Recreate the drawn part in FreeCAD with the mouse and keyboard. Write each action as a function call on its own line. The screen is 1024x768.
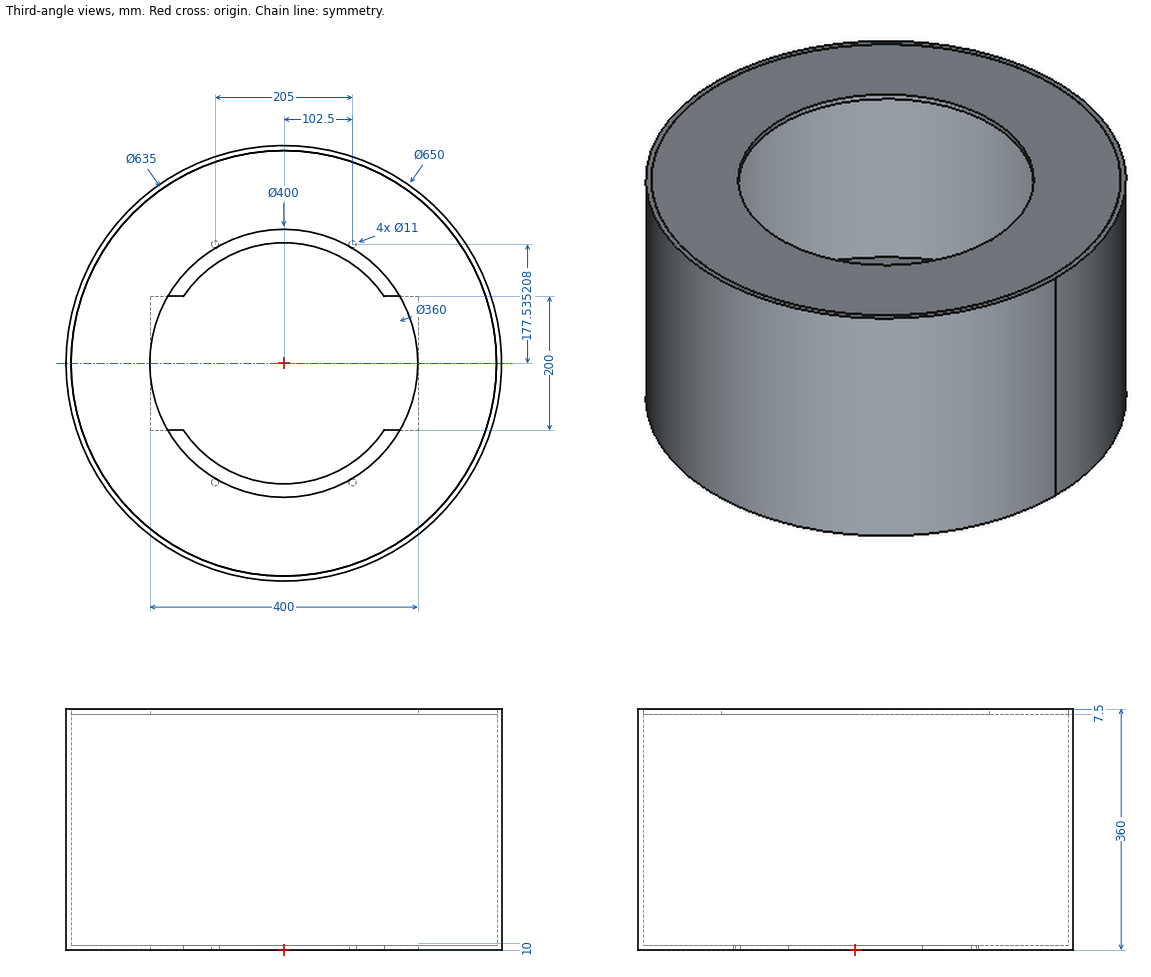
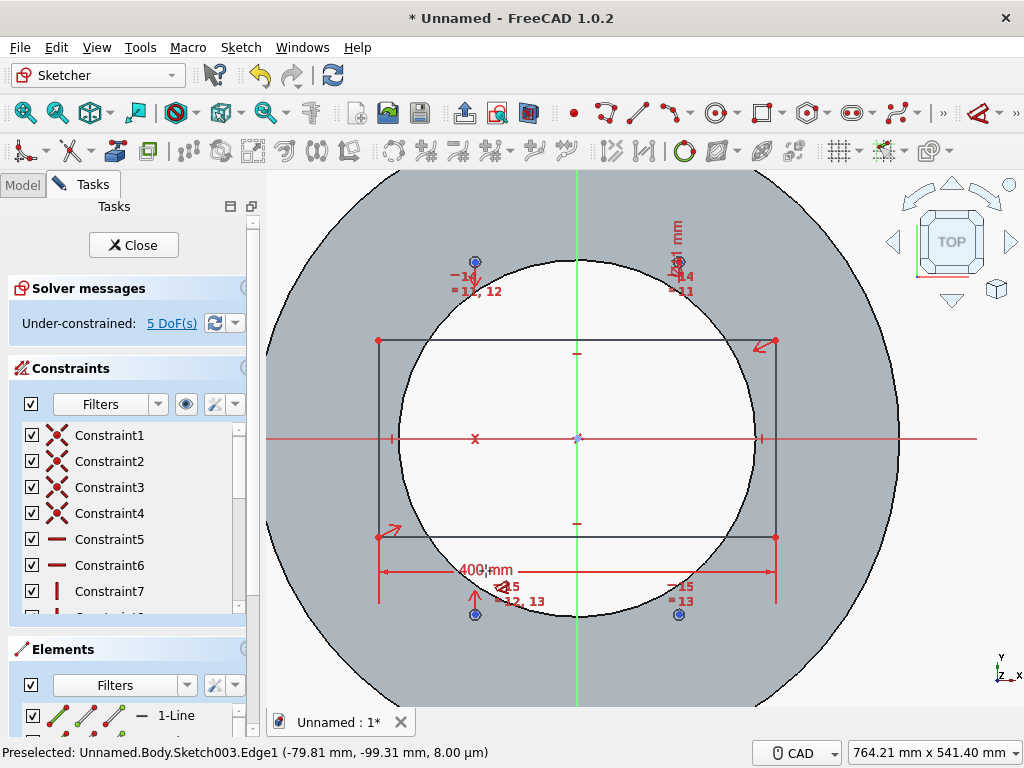
click(776, 478)
click(810, 393)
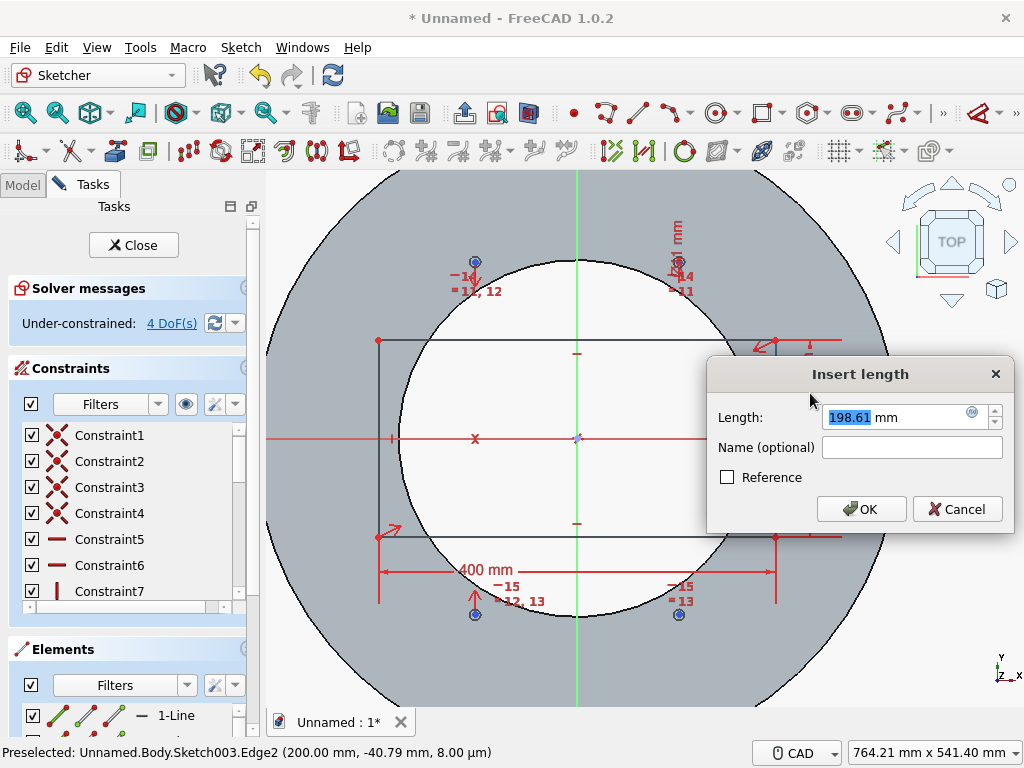
text(200)
key(Return)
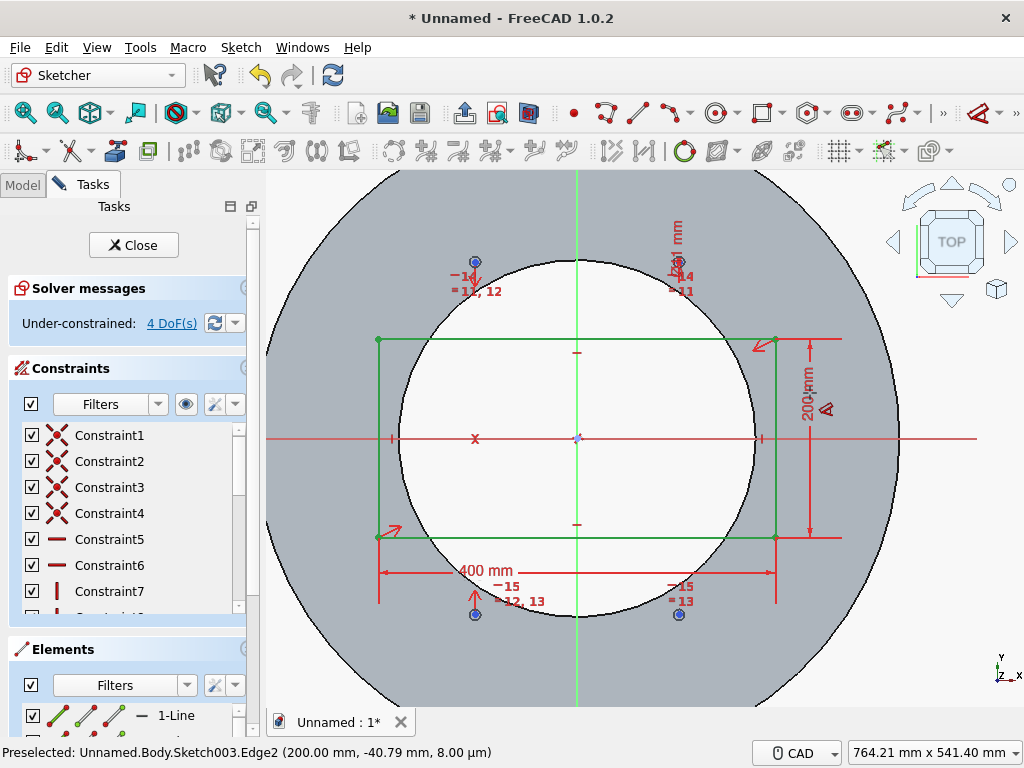
click(679, 262)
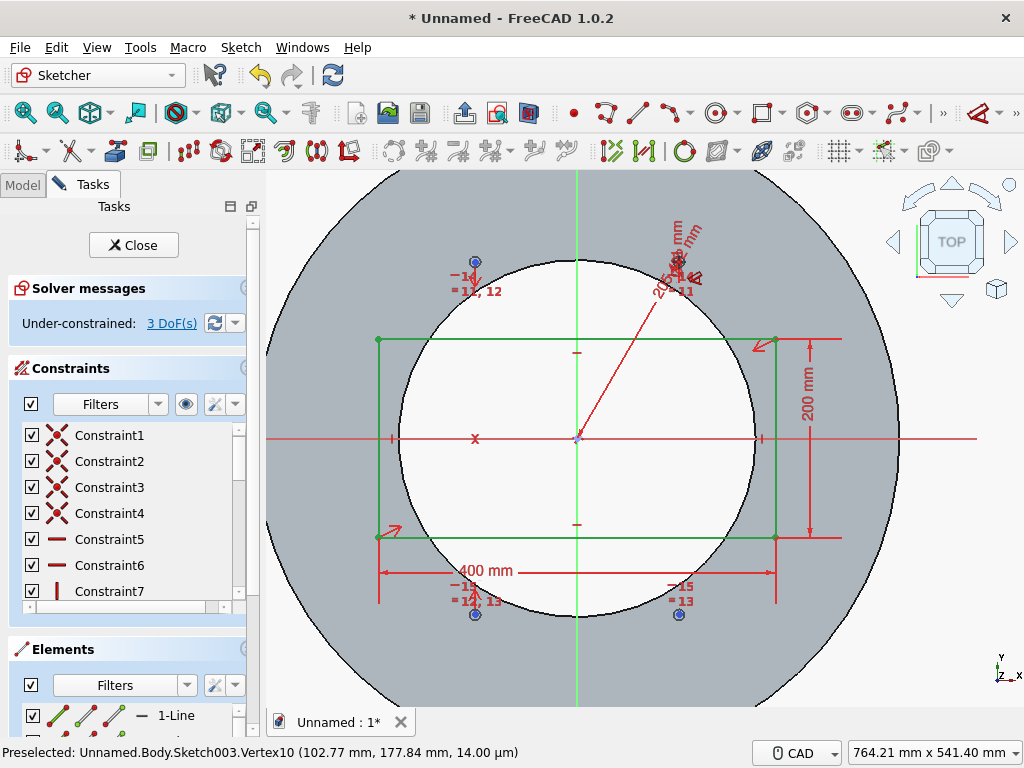
click(475, 262)
click(530, 228)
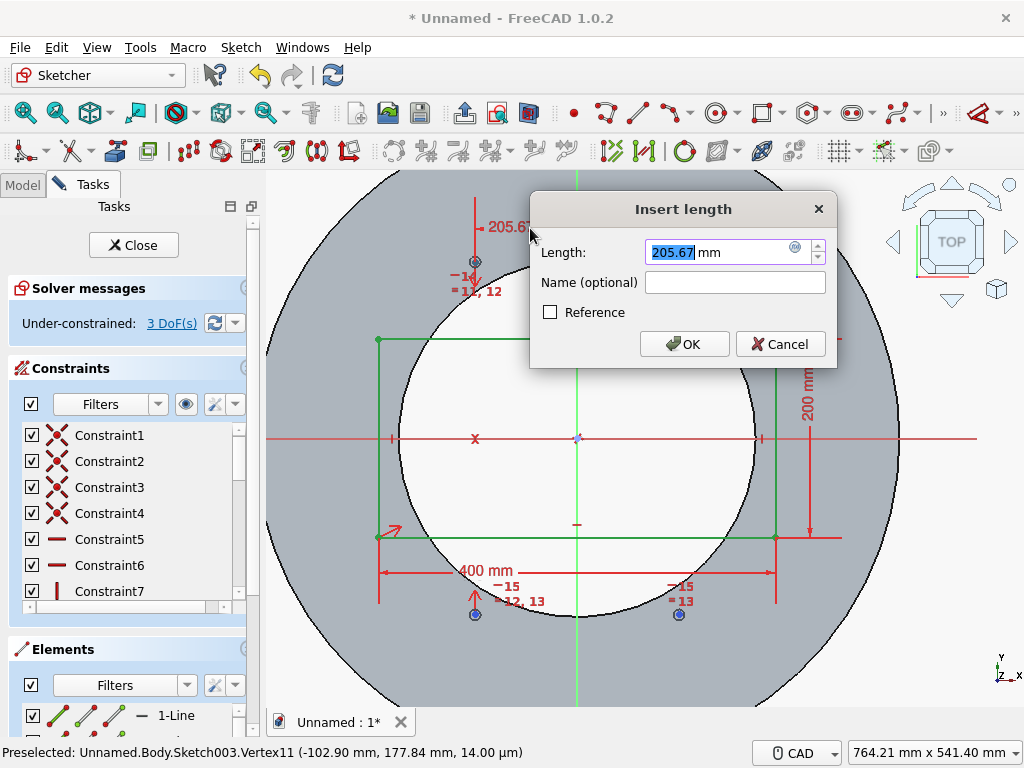
text(205)
key(Return)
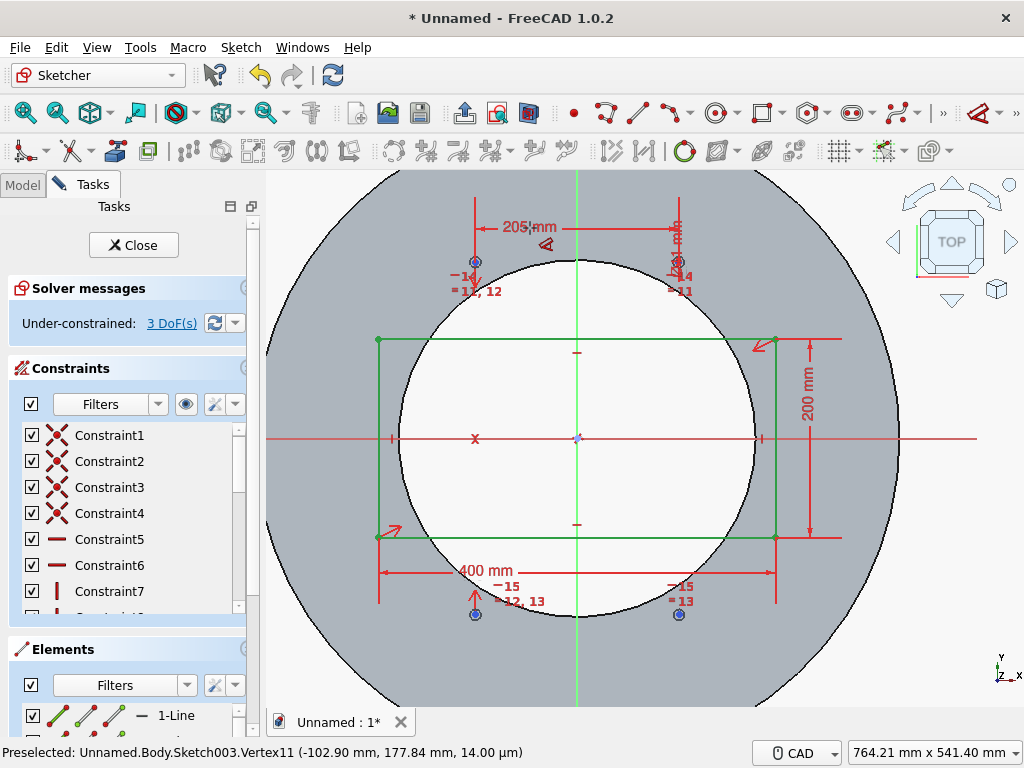
click(475, 615)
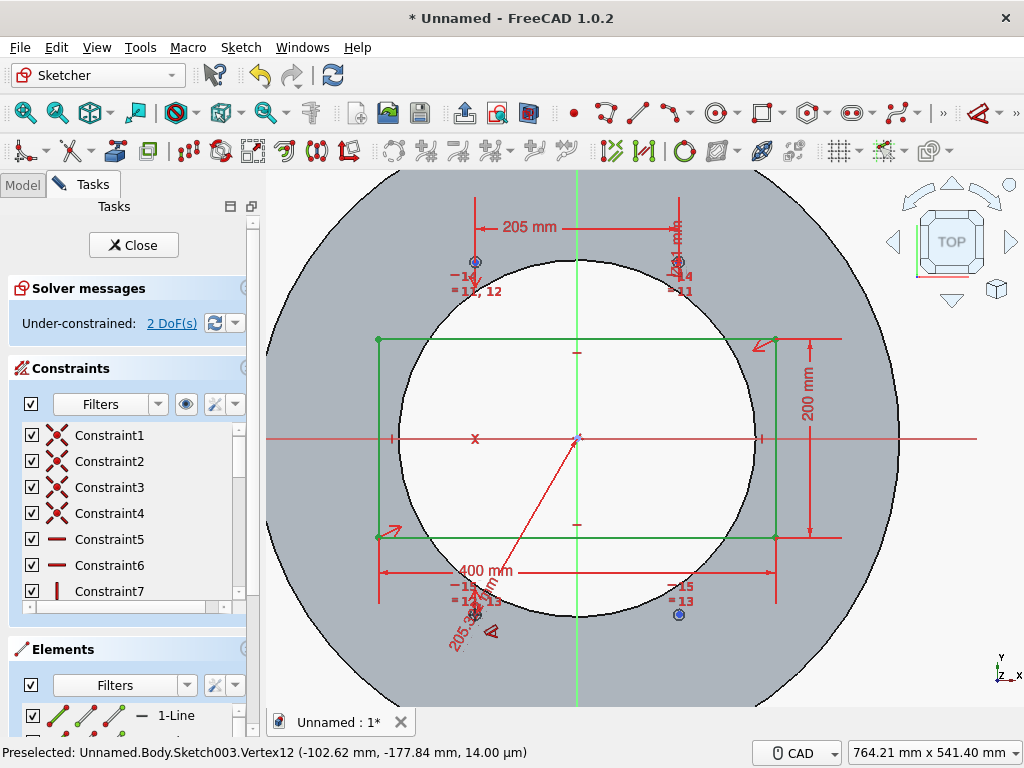
click(679, 615)
click(530, 649)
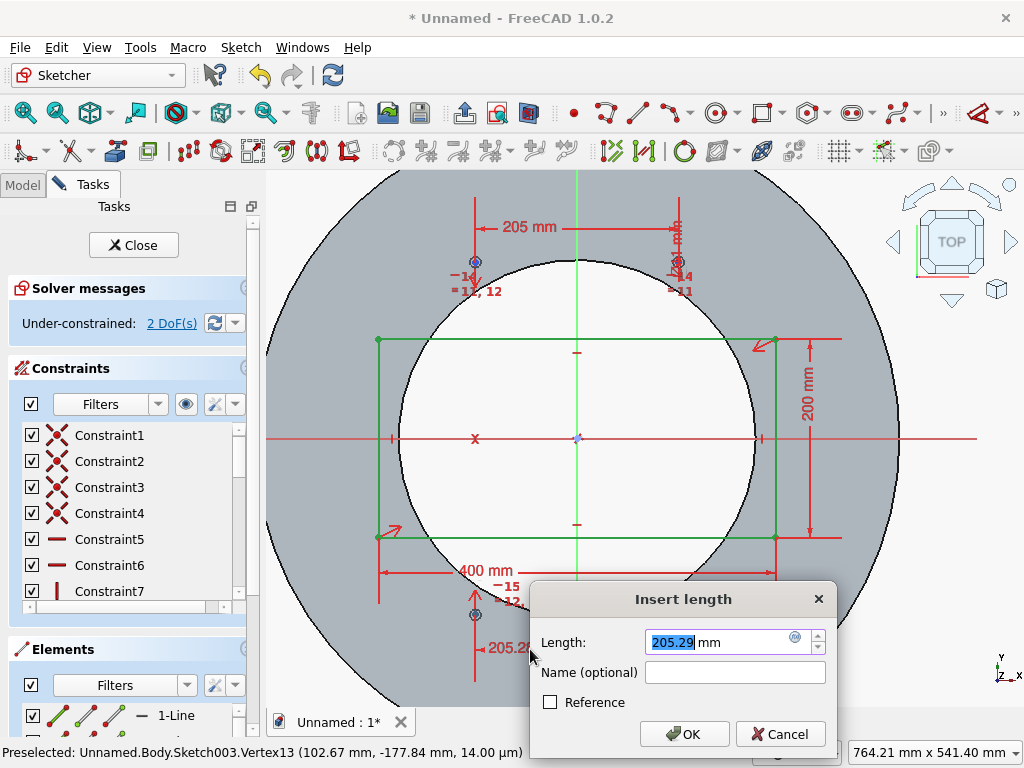
text(205)
key(Return)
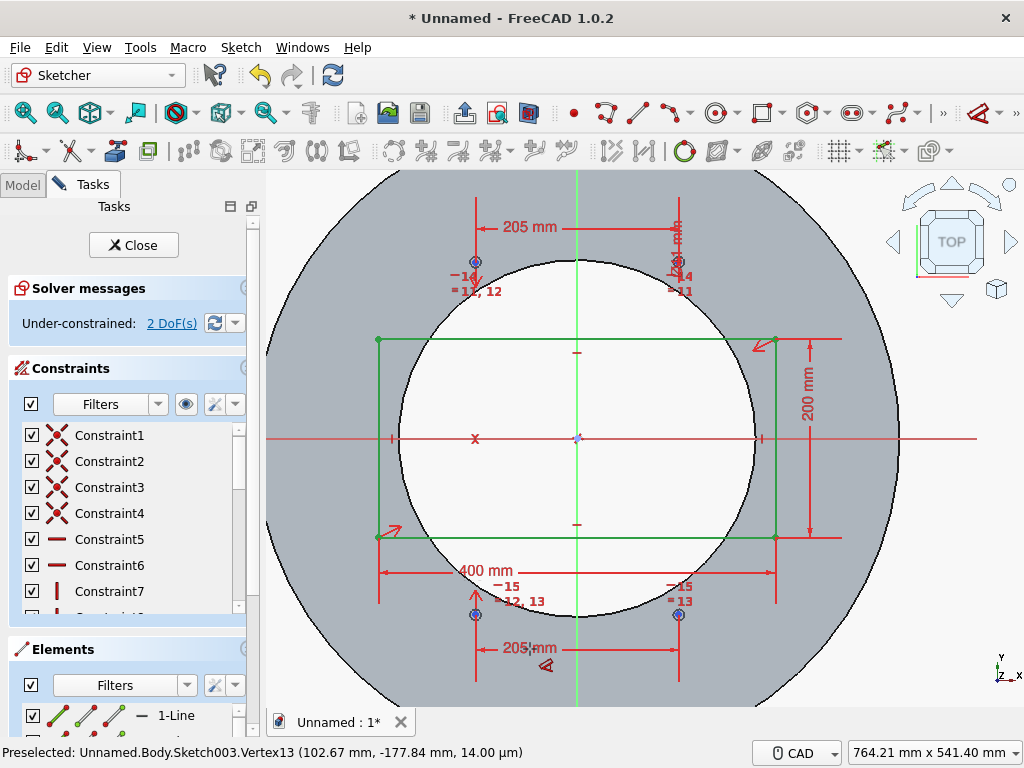
click(679, 262)
click(628, 228)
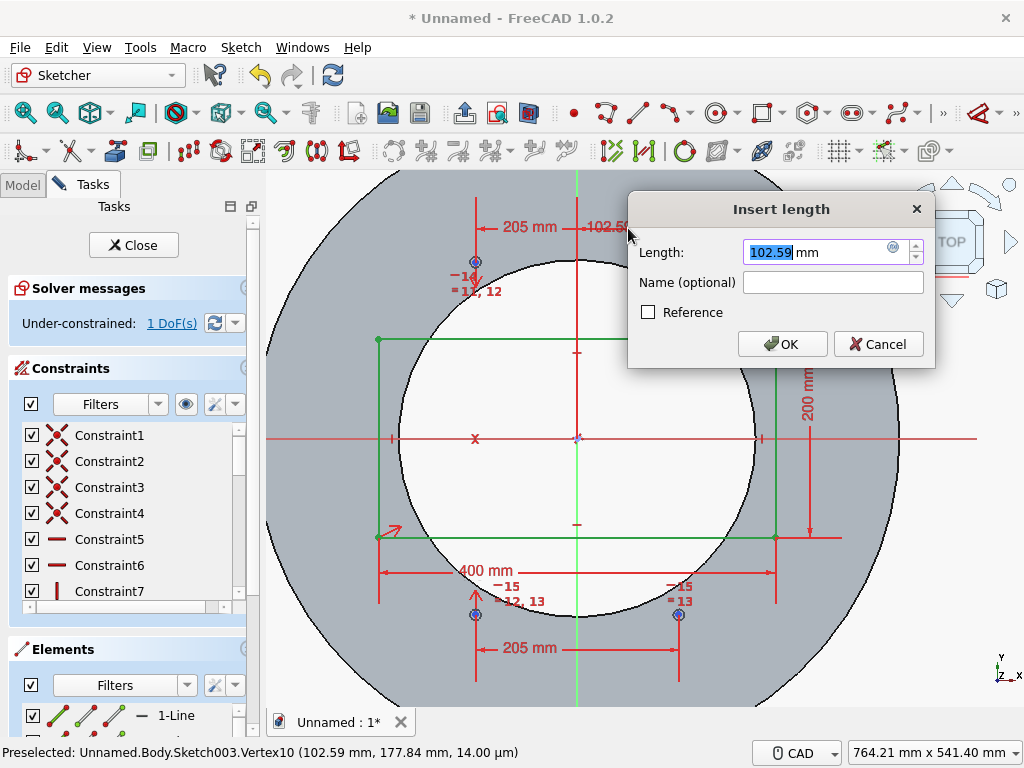
text(102.5)
key(Return)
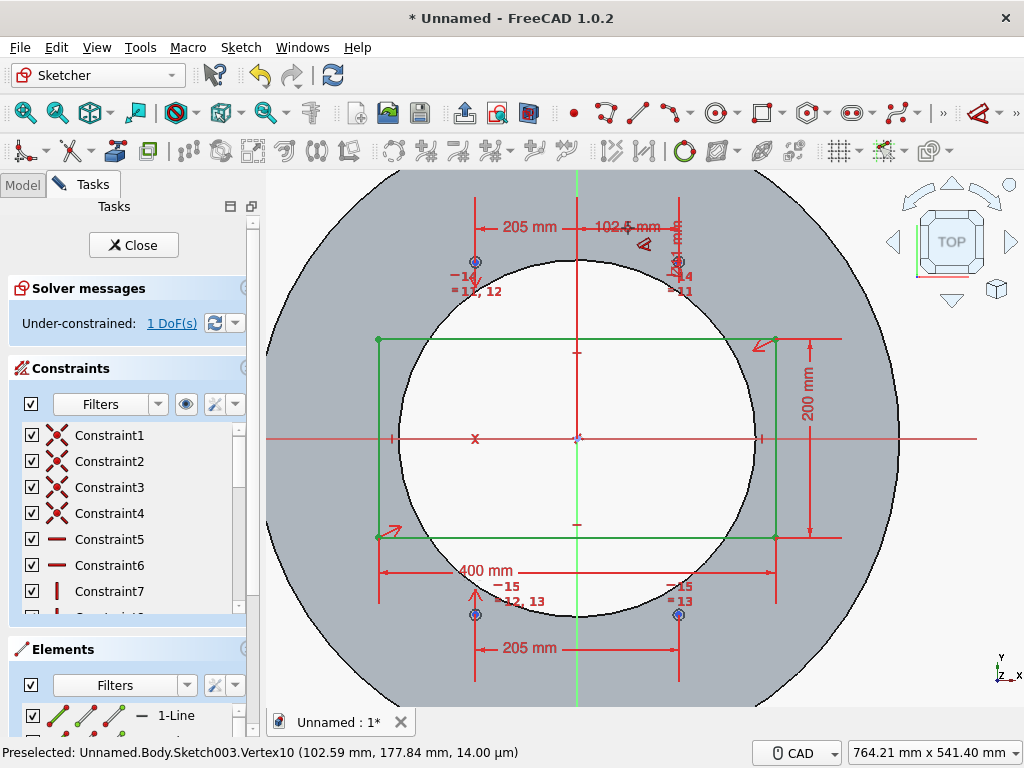
click(679, 262)
click(713, 310)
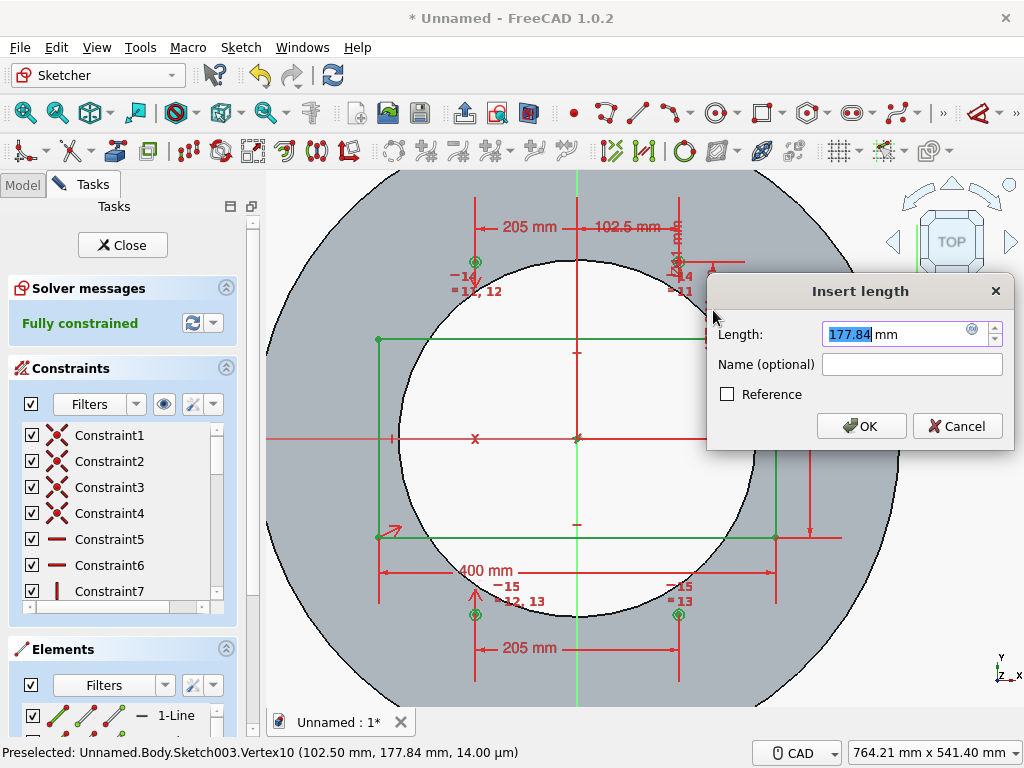
text(177.535208)
key(Return)
key(Escape)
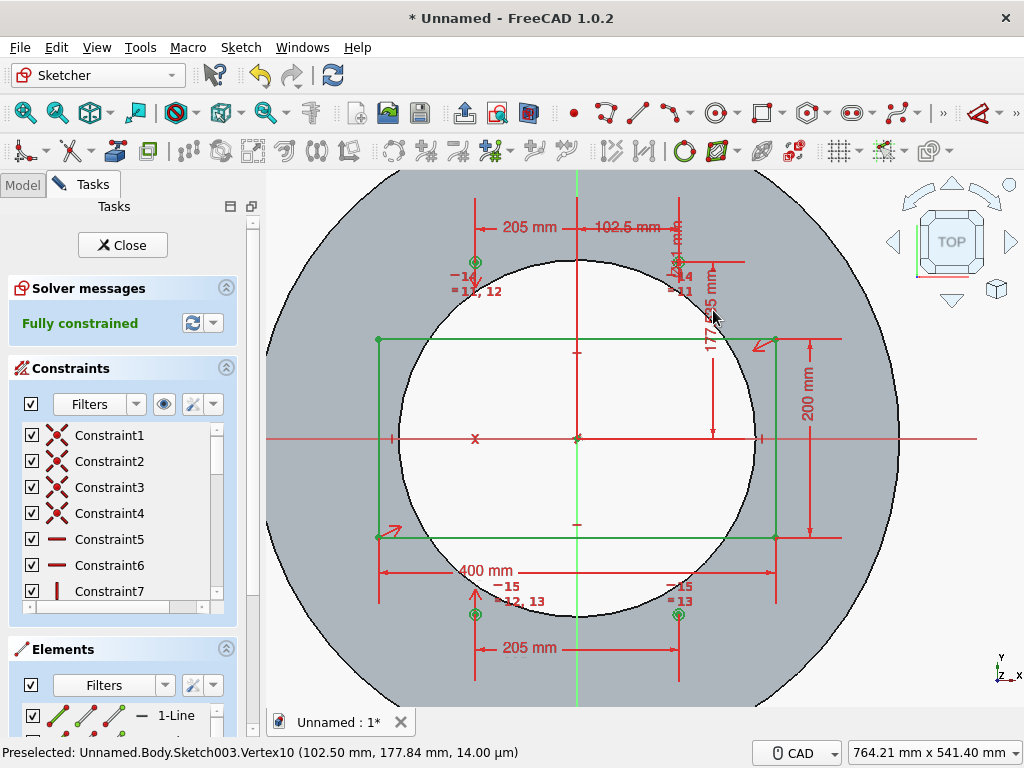
click(123, 245)